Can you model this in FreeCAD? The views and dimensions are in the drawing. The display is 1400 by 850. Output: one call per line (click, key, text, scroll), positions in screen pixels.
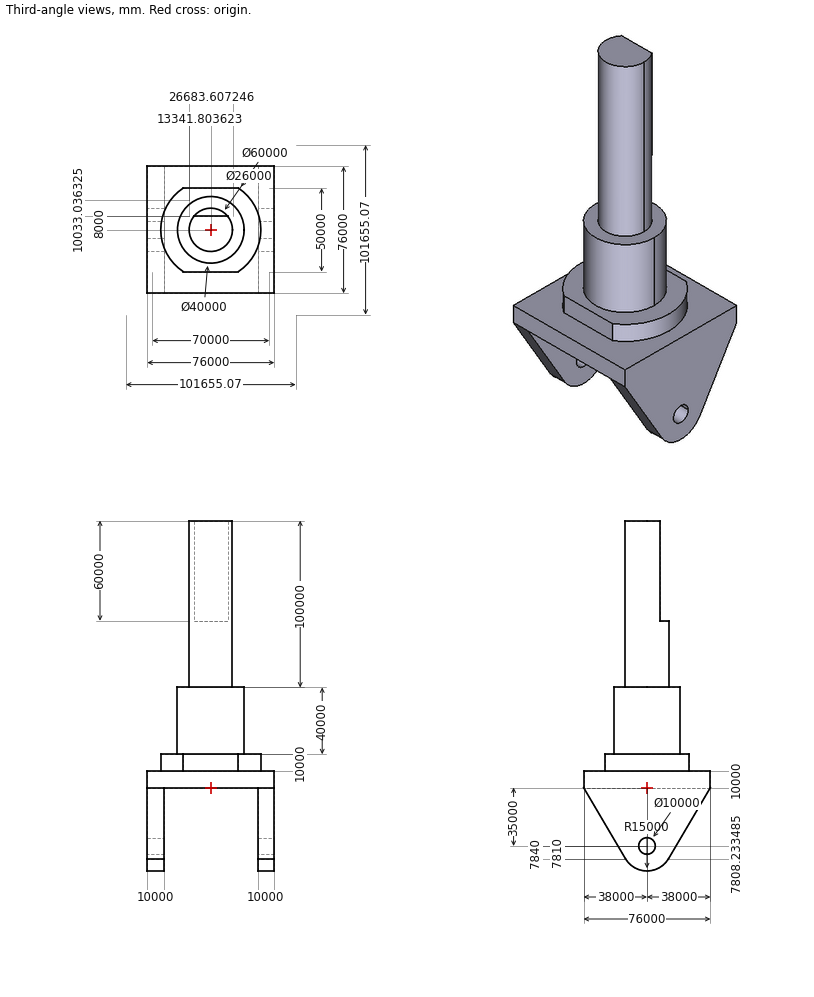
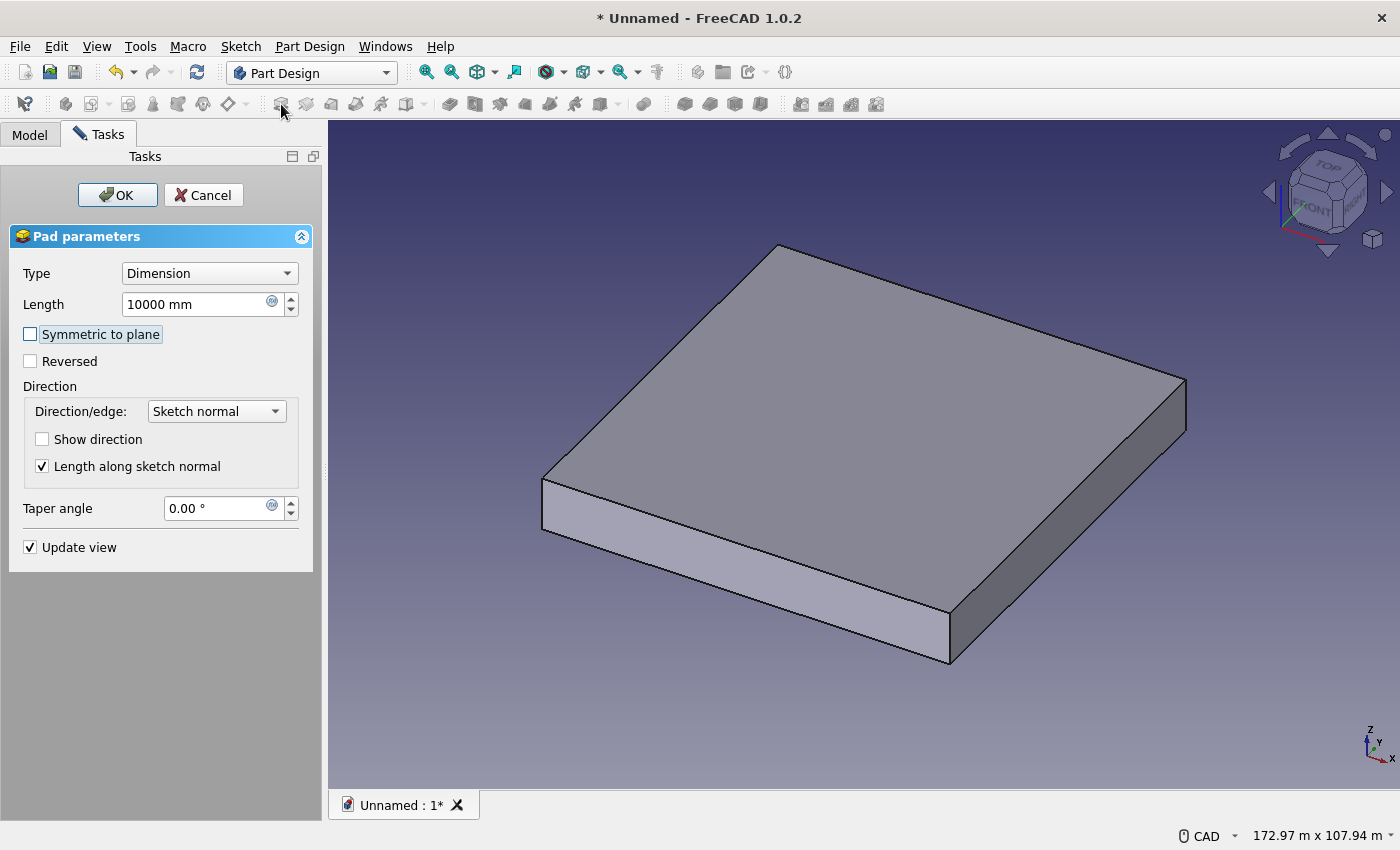
click(31, 361)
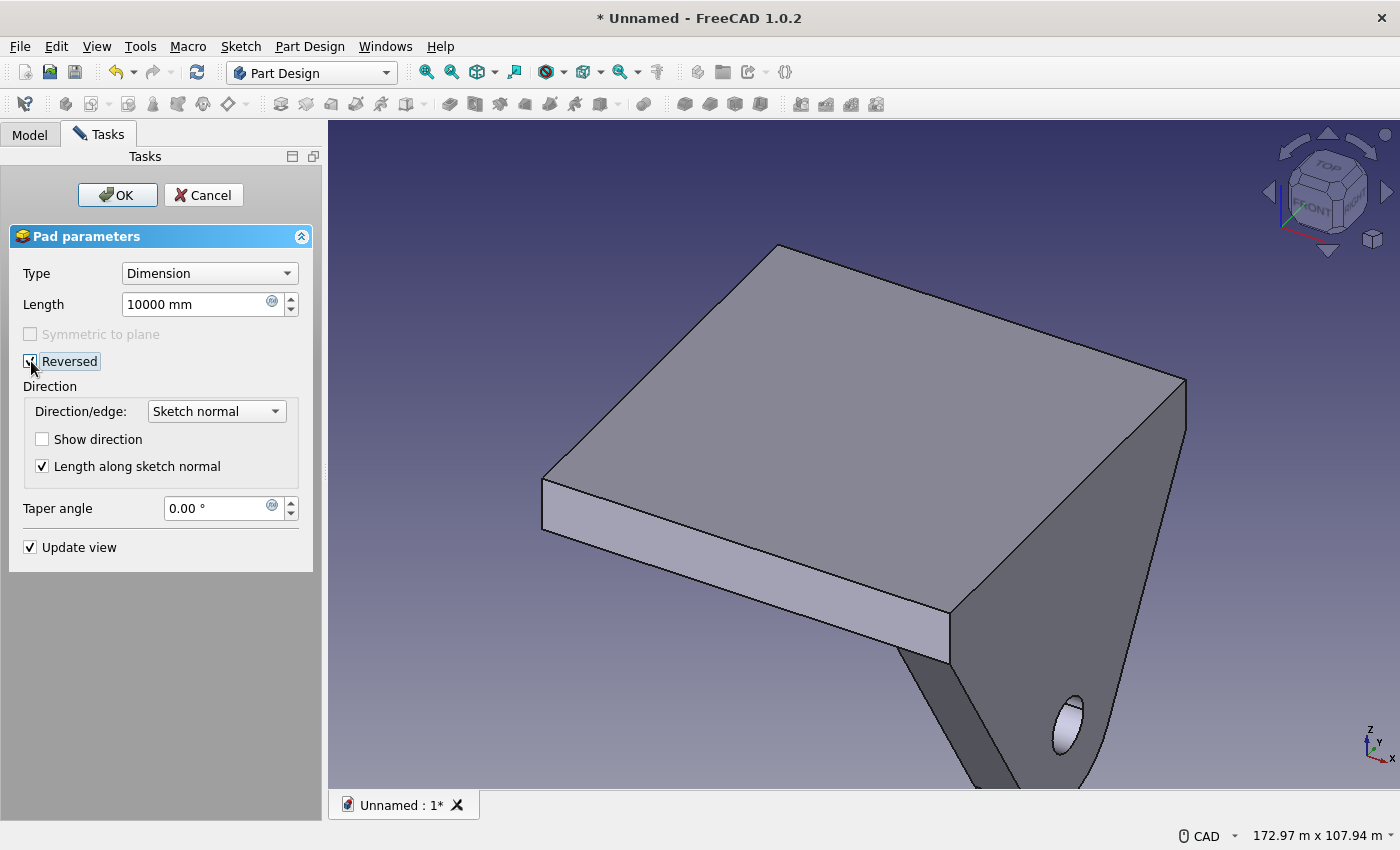
click(118, 195)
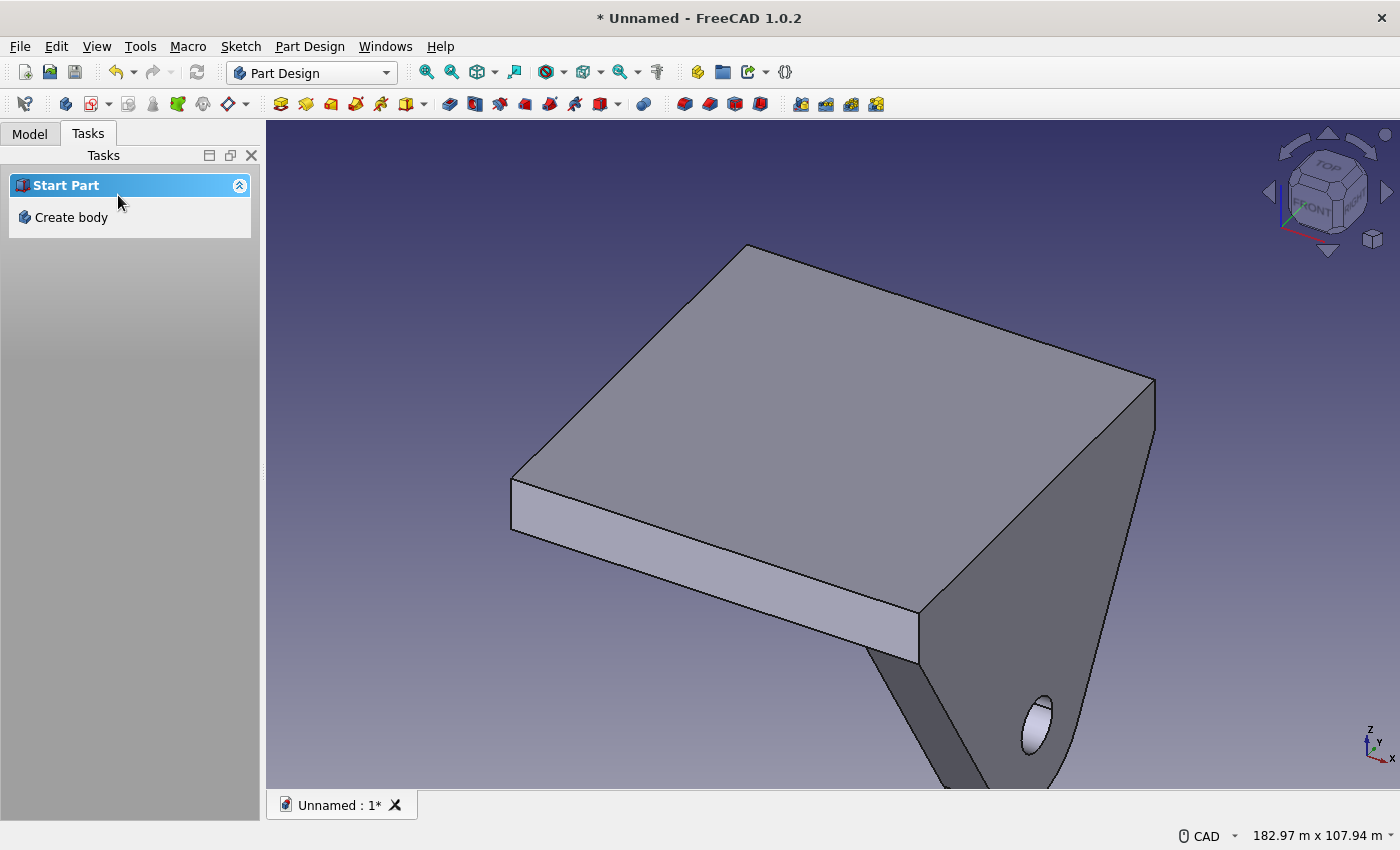
click(427, 72)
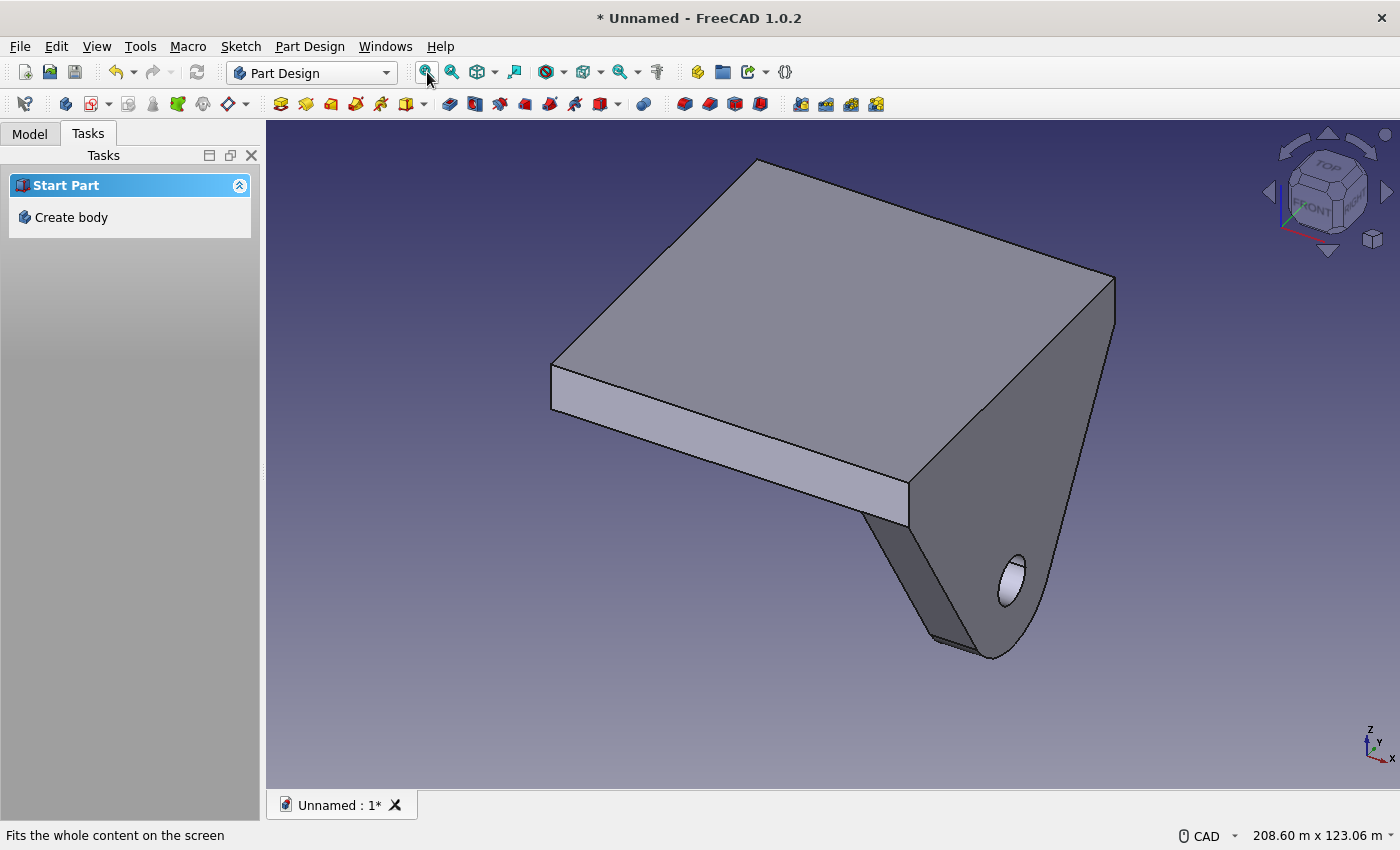
click(30, 134)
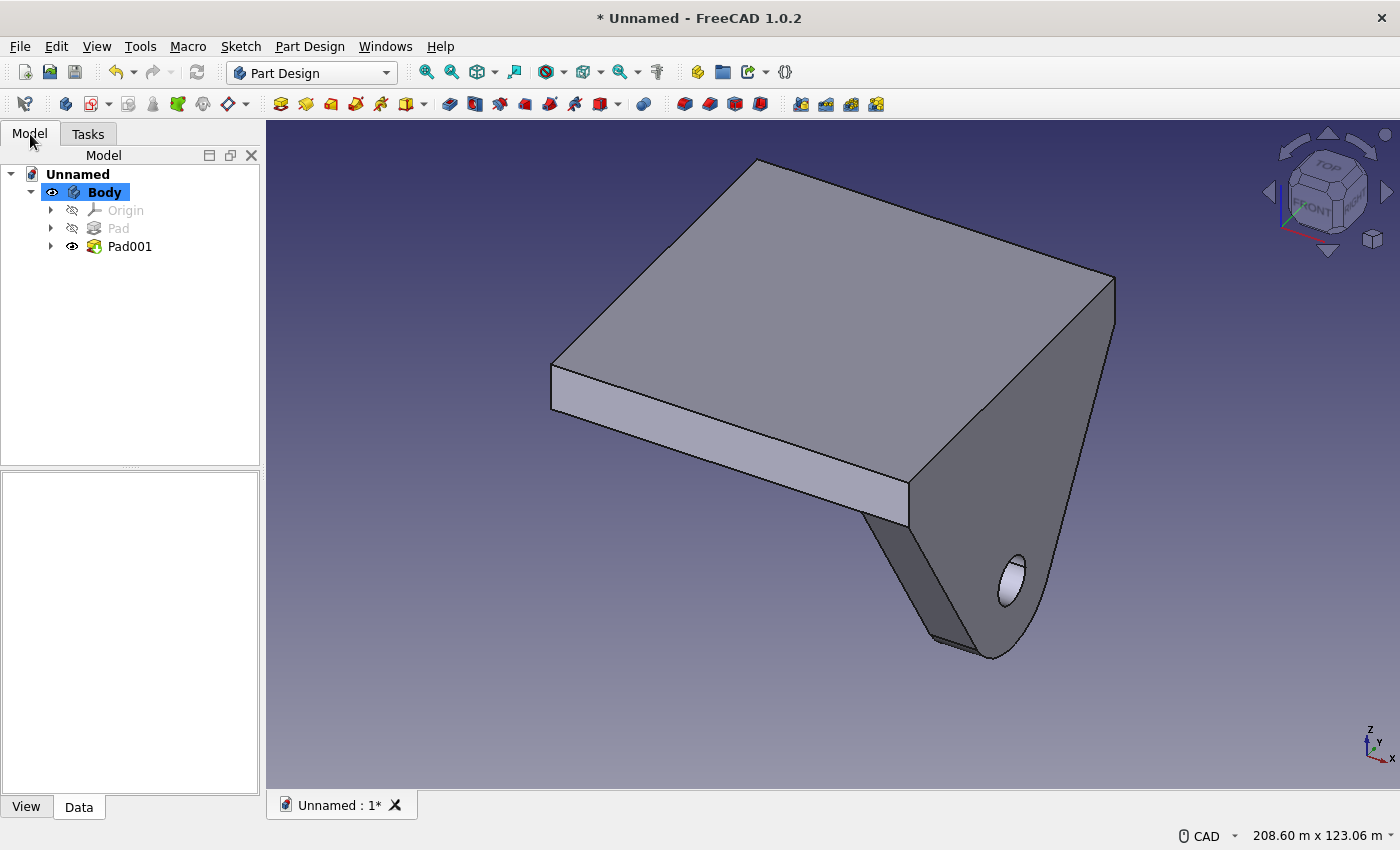
click(51, 210)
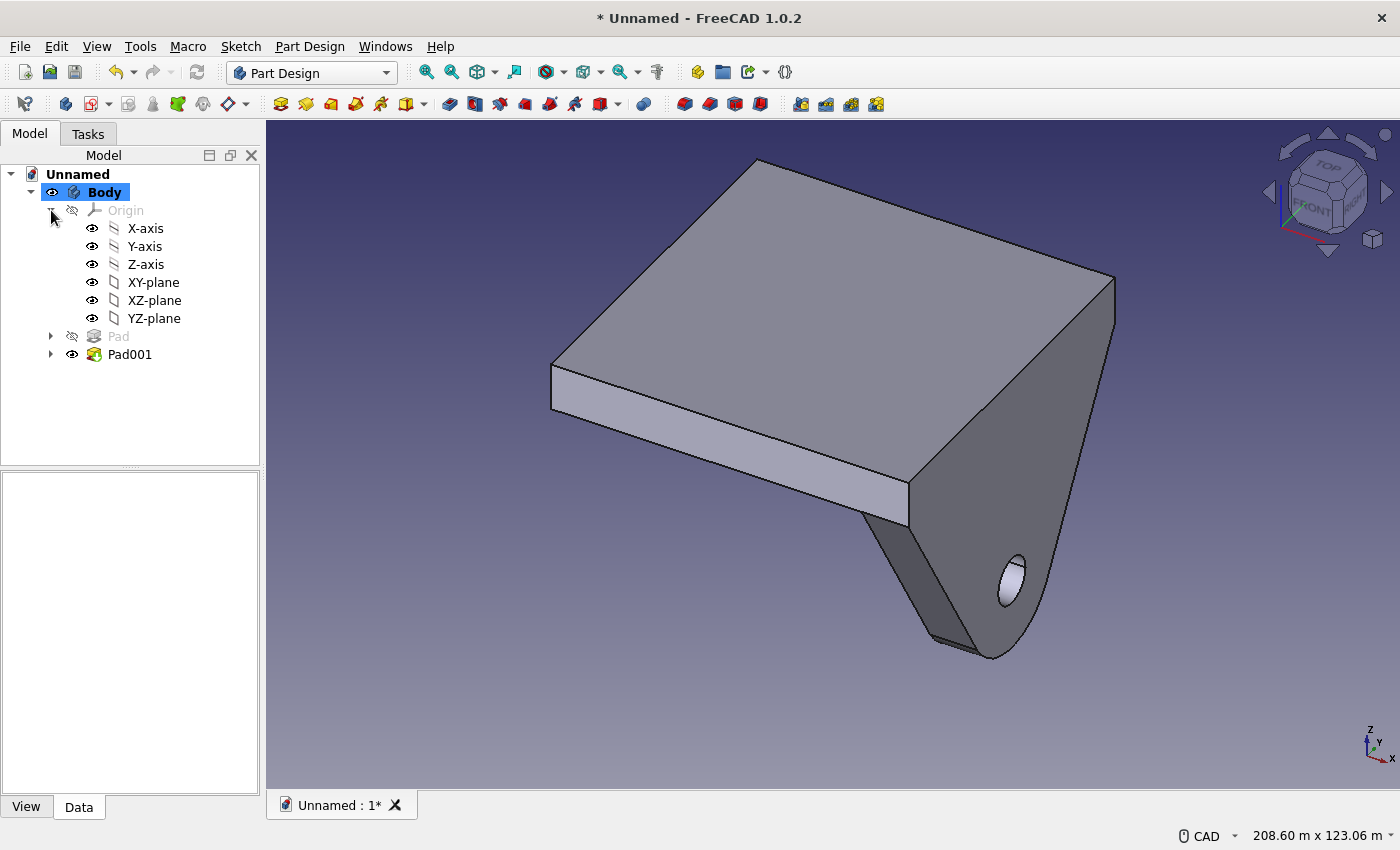
click(137, 318)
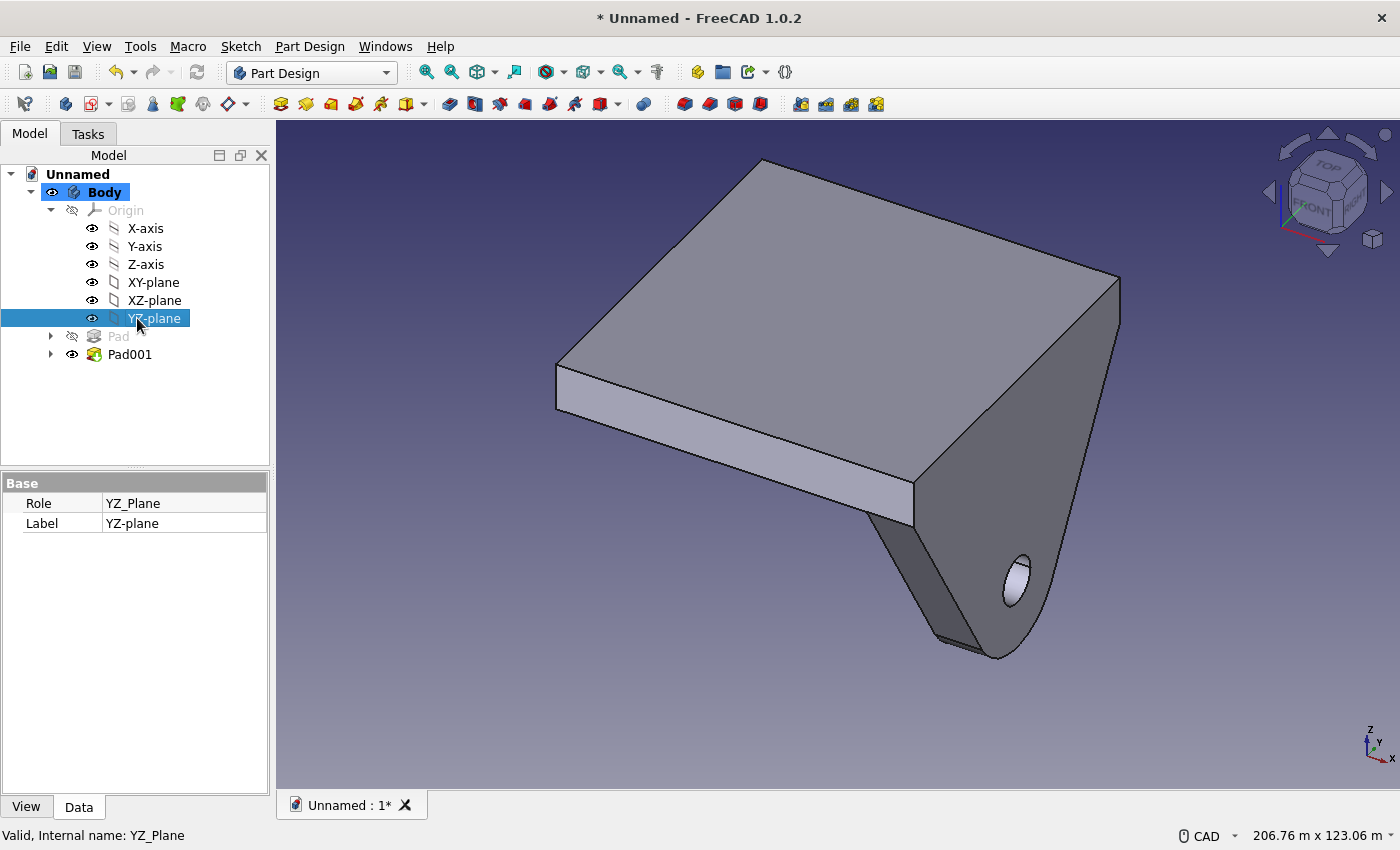
click(228, 104)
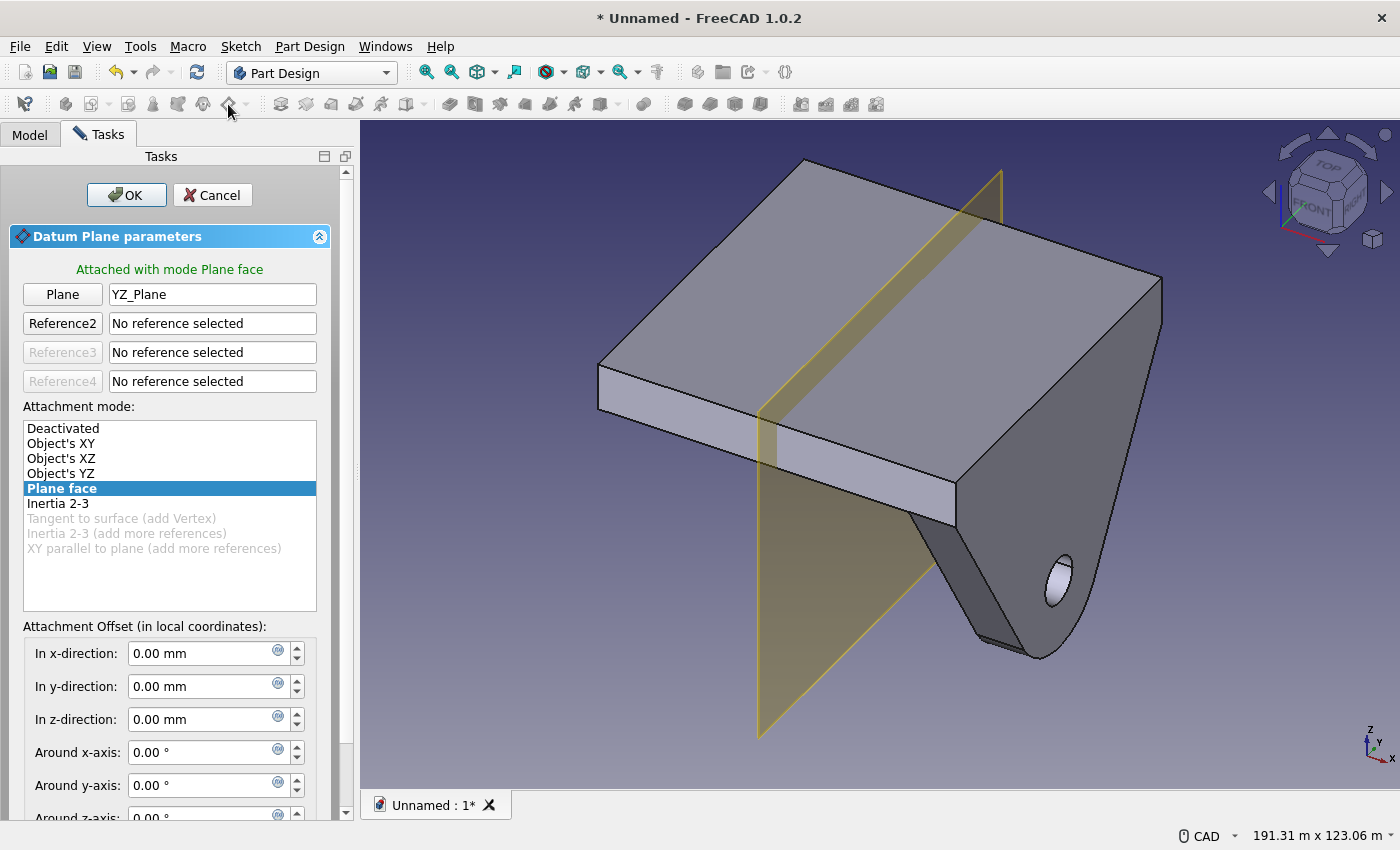
triple_click(210, 720)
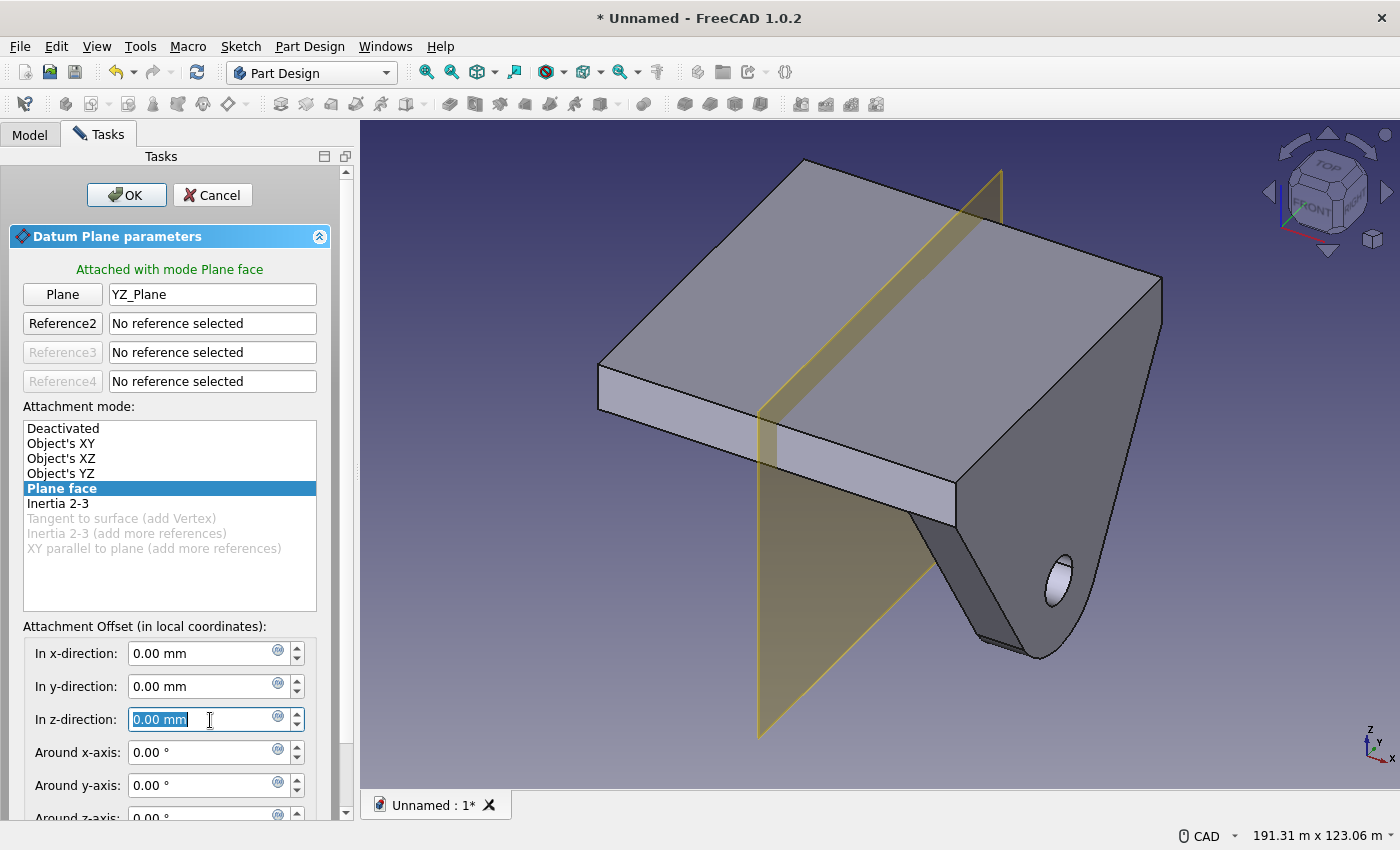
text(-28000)
key(Tab)